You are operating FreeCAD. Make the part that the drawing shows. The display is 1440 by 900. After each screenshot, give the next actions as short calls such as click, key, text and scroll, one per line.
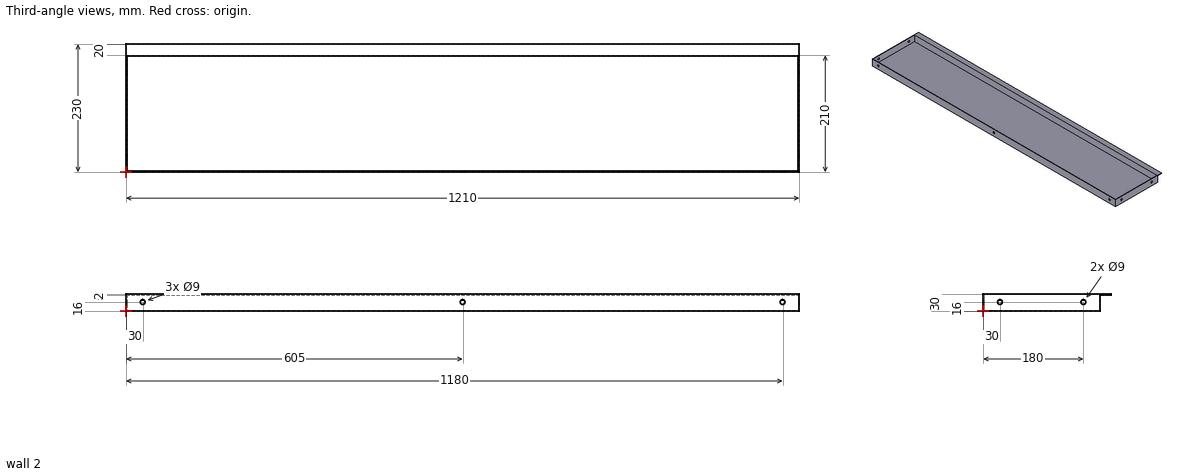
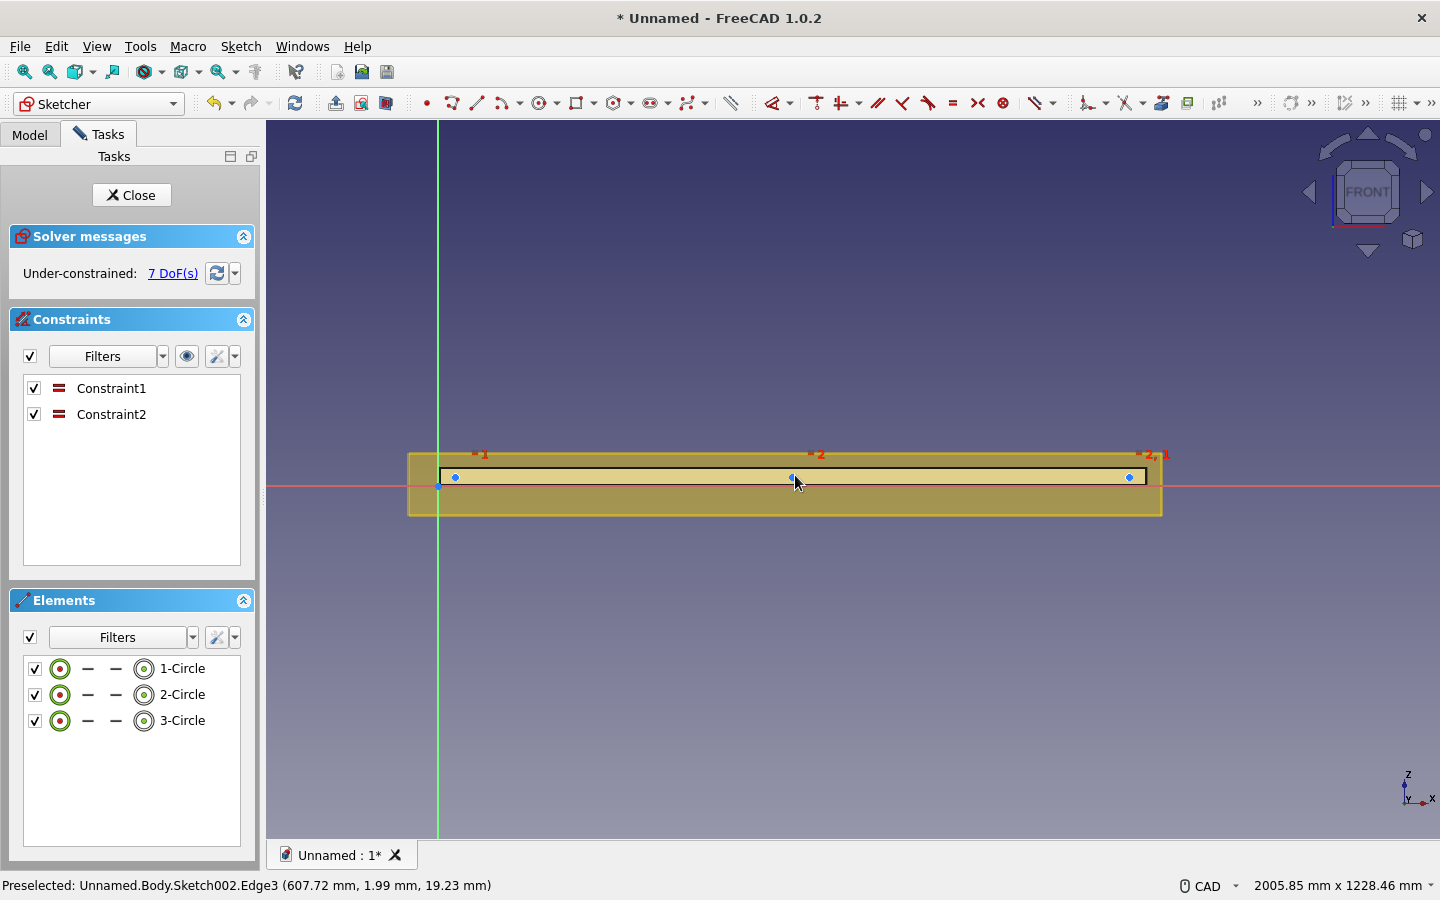
click(456, 477)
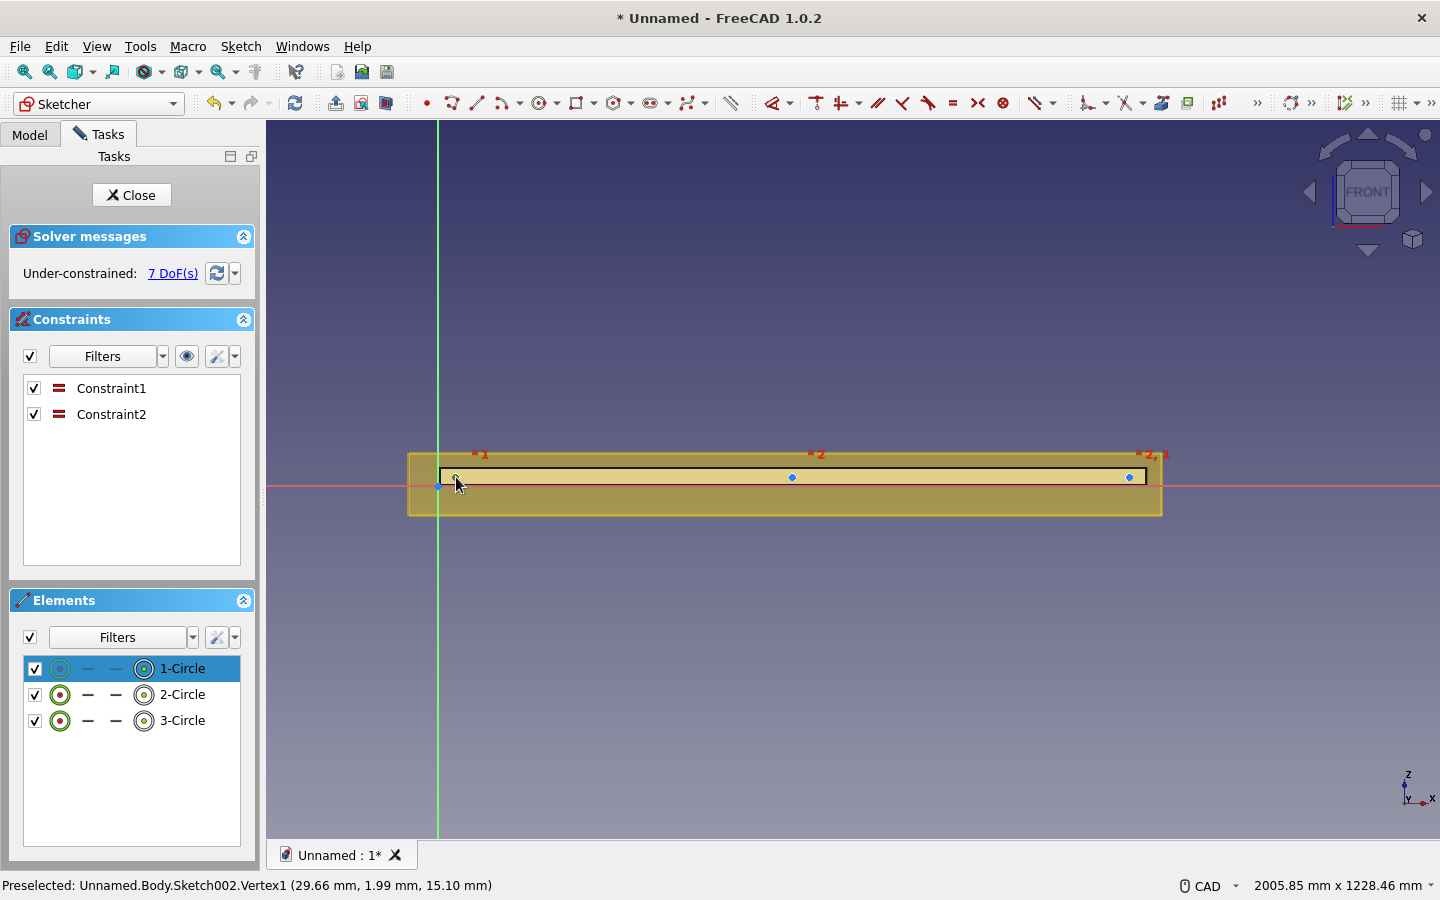
click(1129, 477)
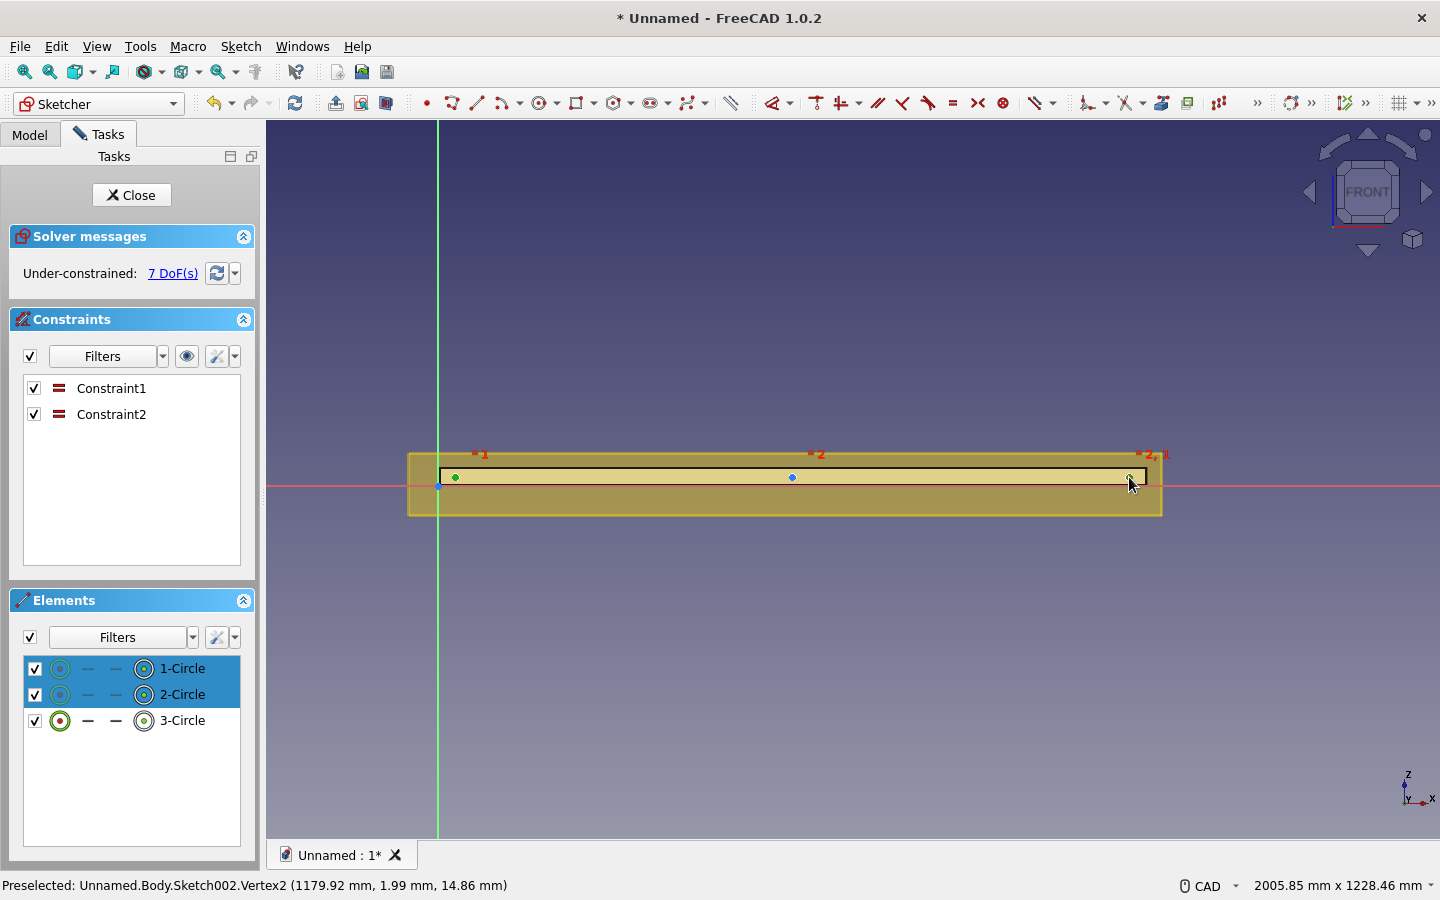
click(858, 104)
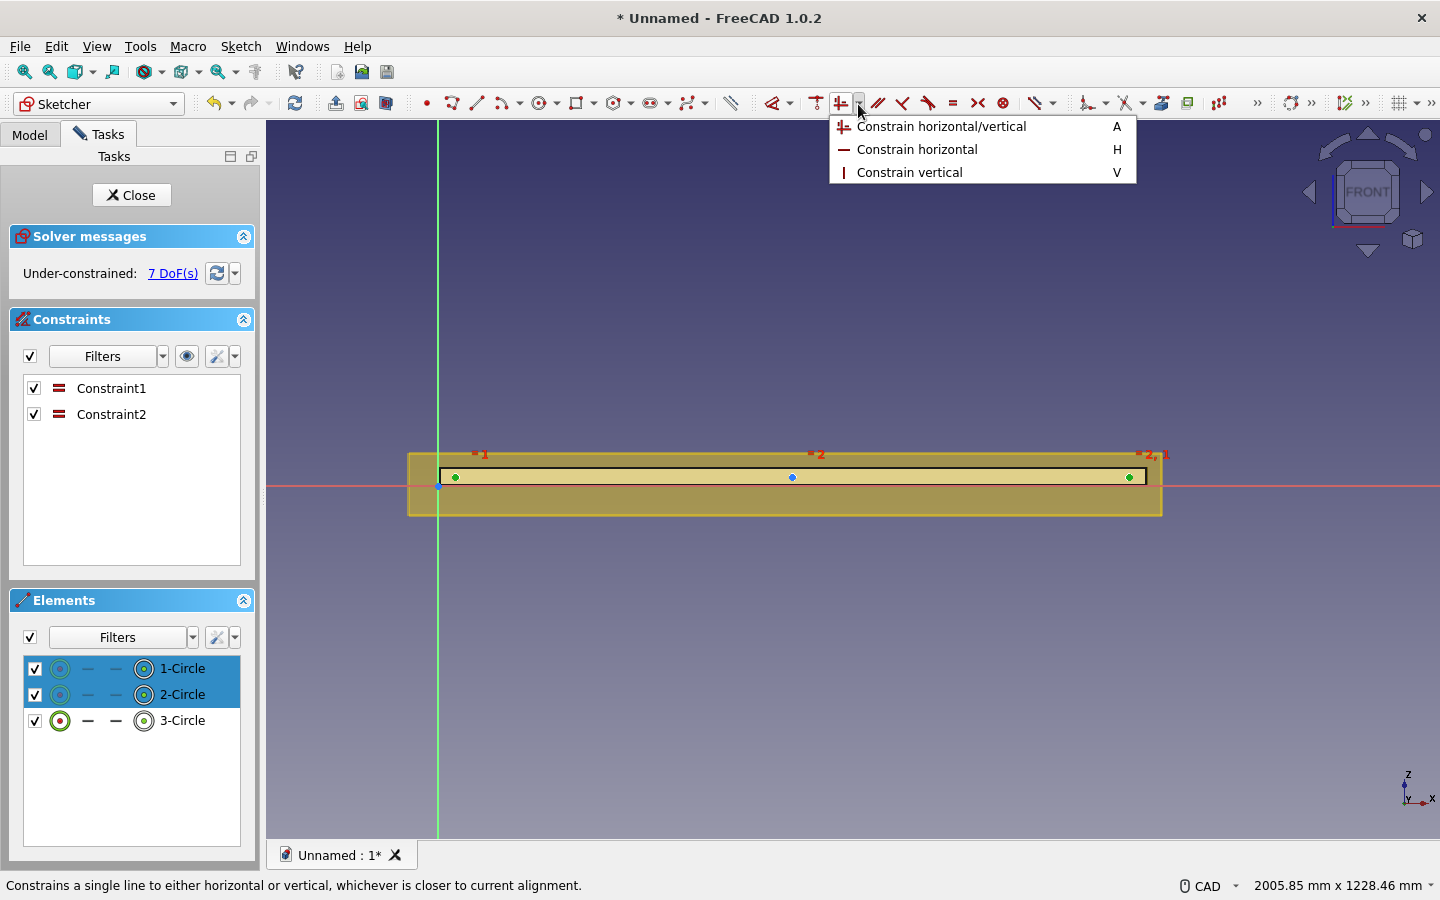
click(983, 150)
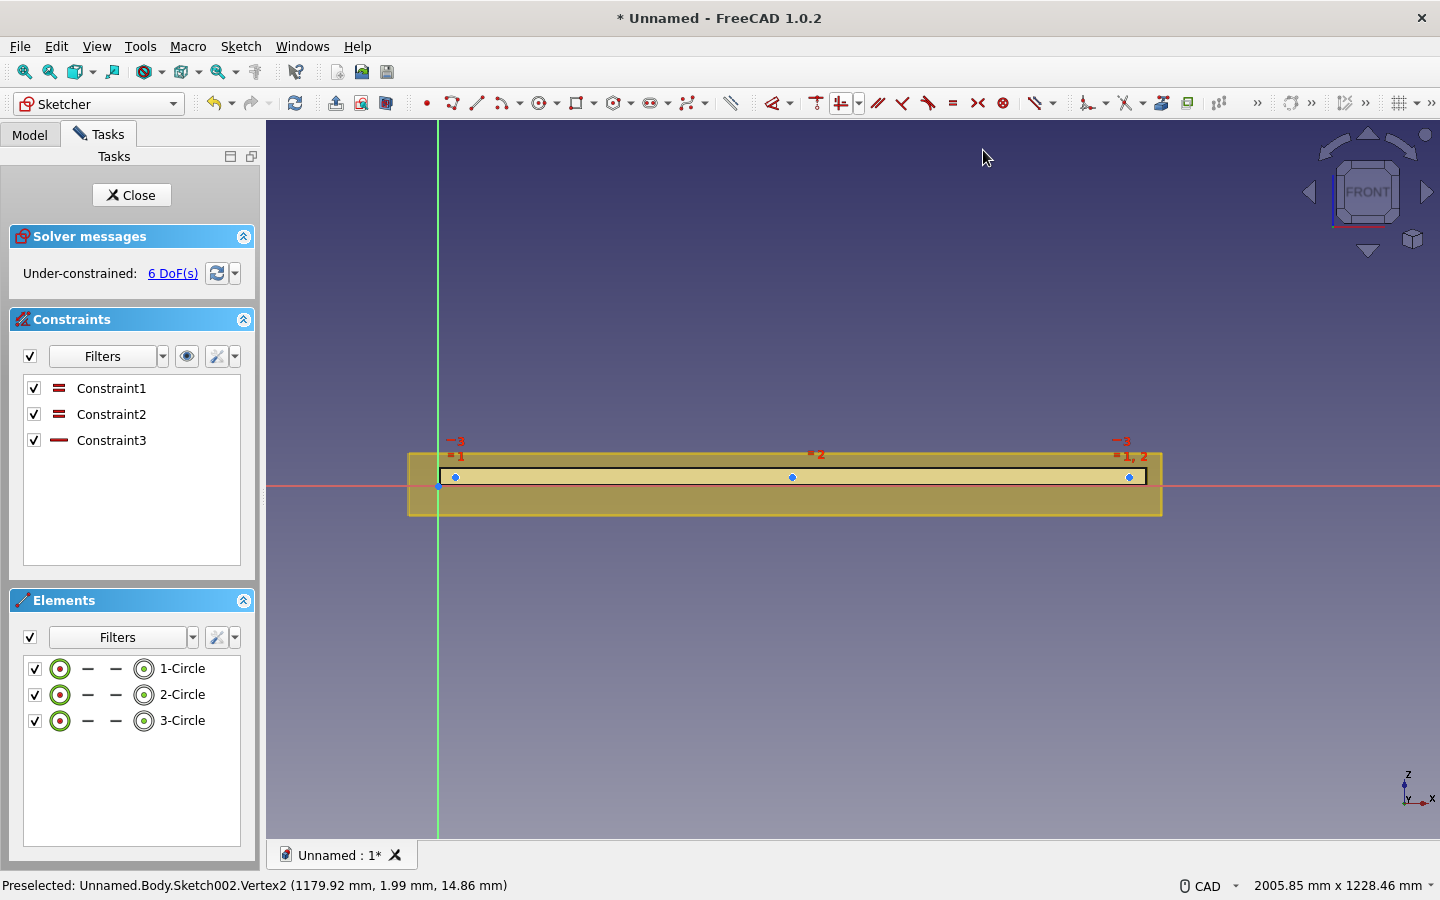
click(456, 477)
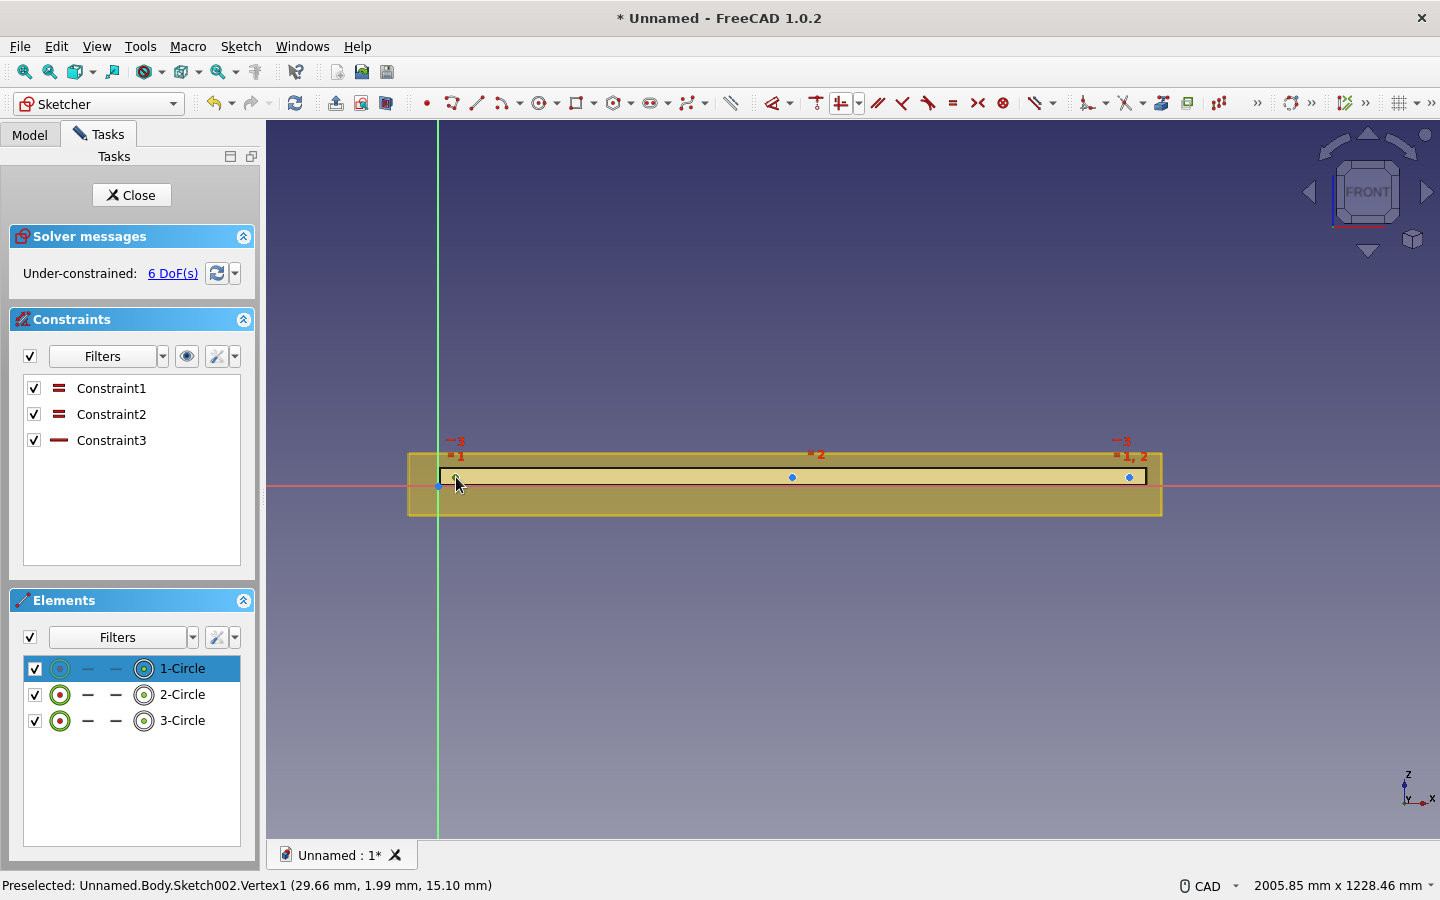
click(793, 477)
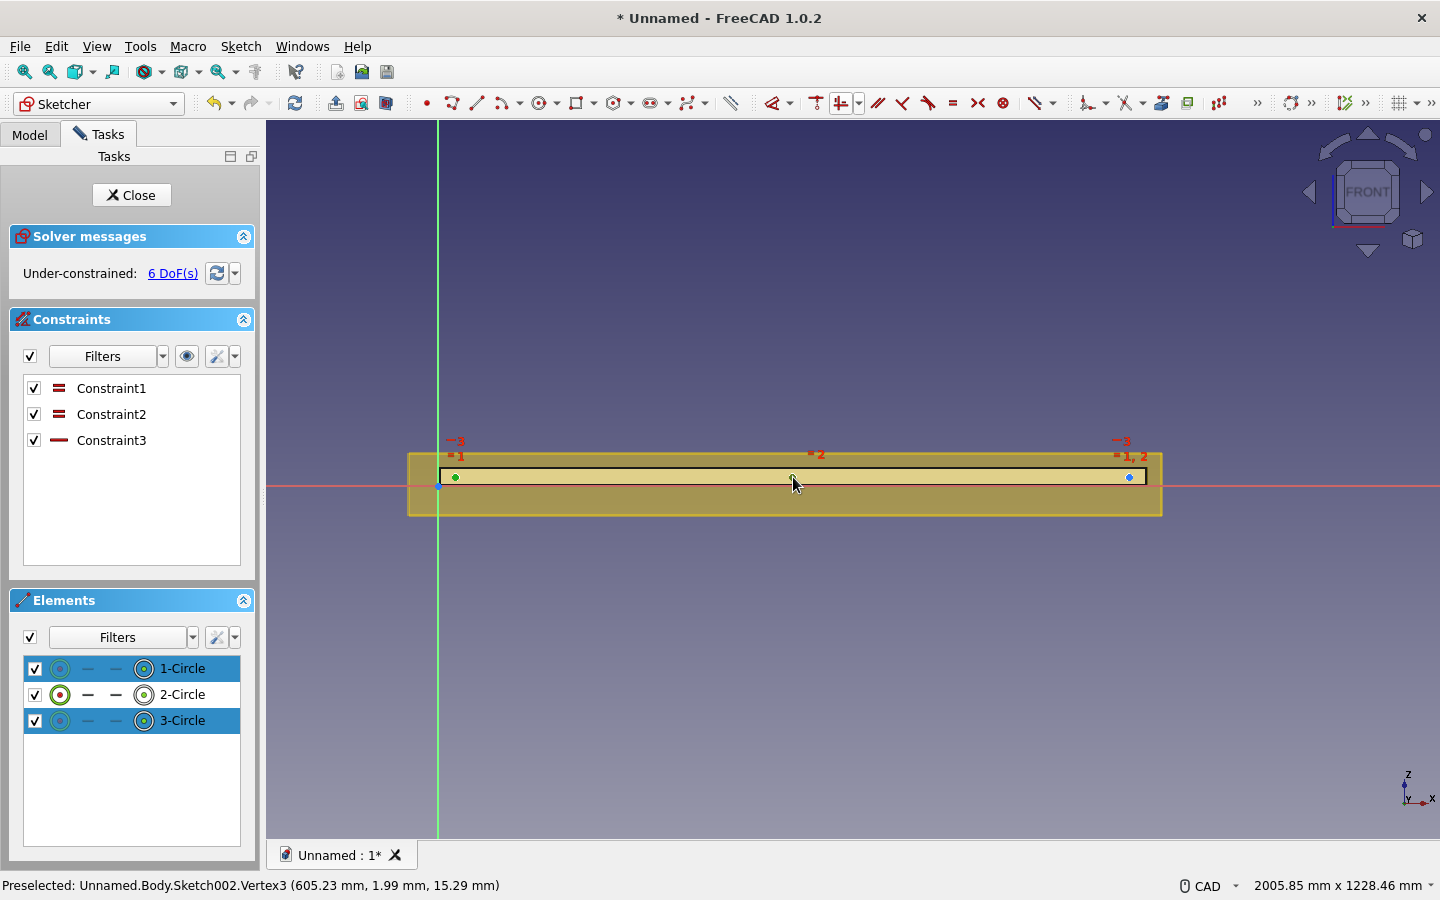
click(858, 104)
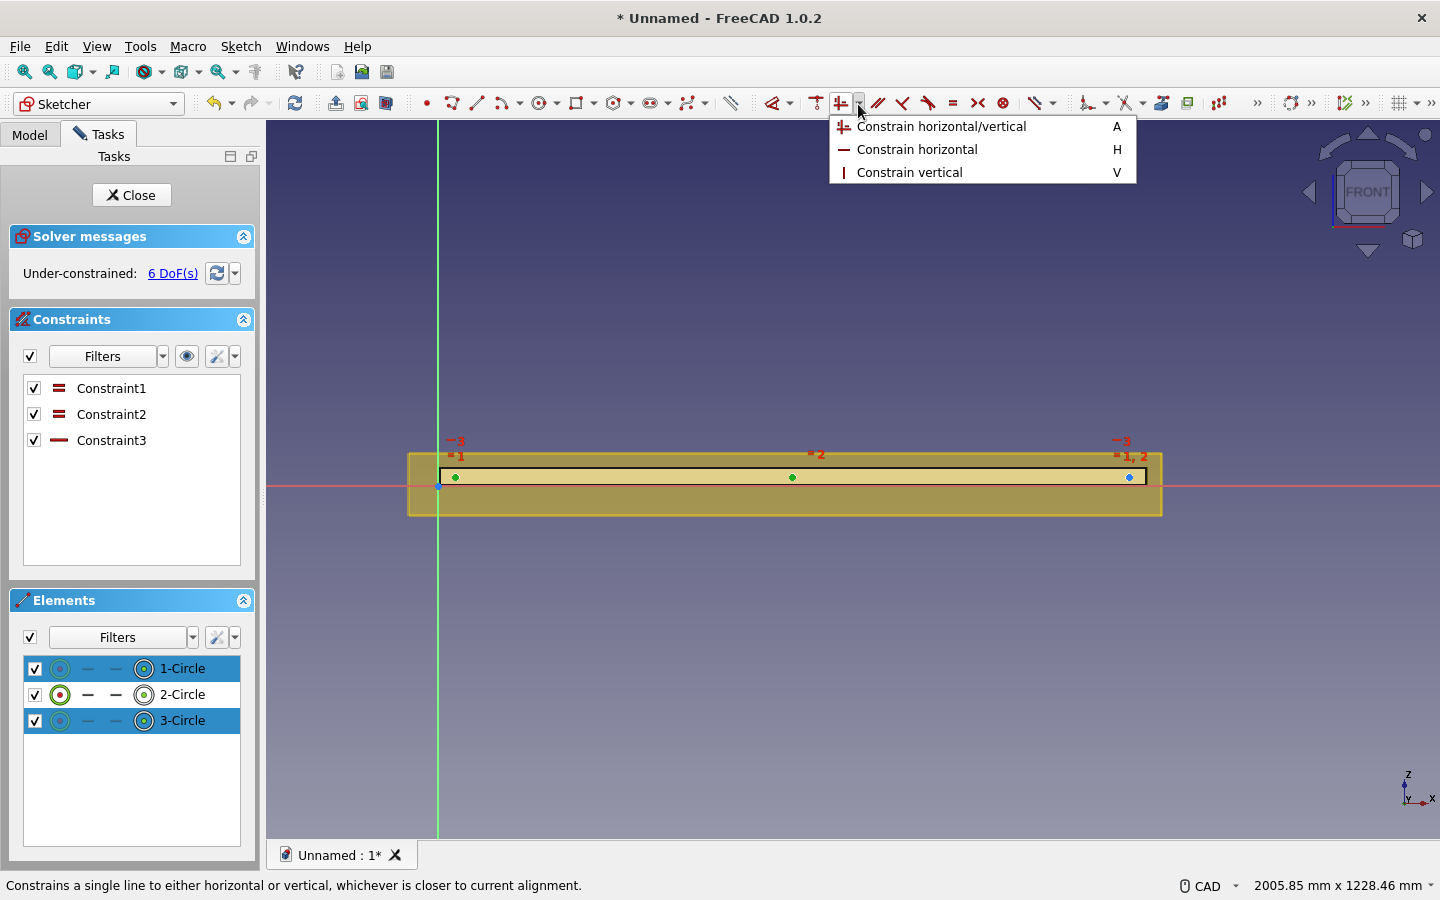
click(983, 150)